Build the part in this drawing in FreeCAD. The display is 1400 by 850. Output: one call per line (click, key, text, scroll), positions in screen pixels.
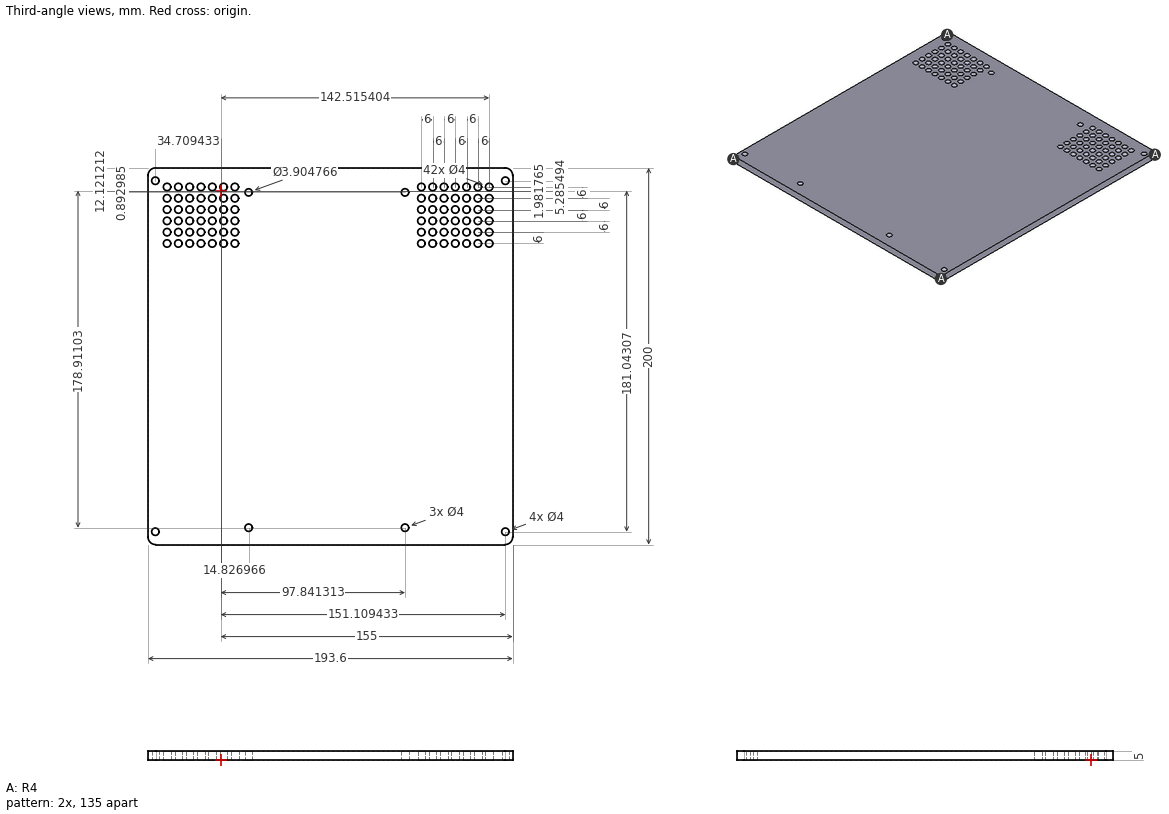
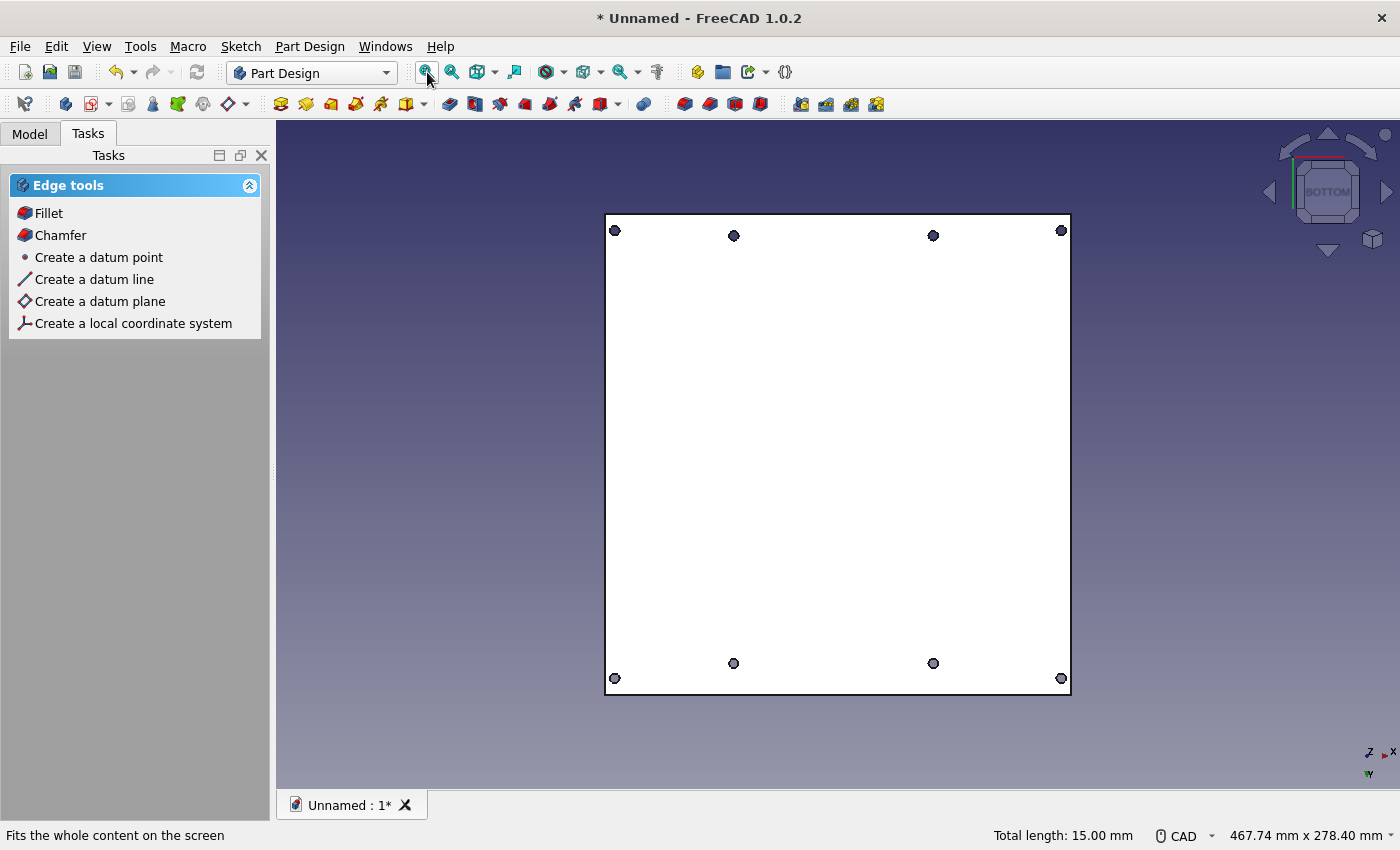
key(4)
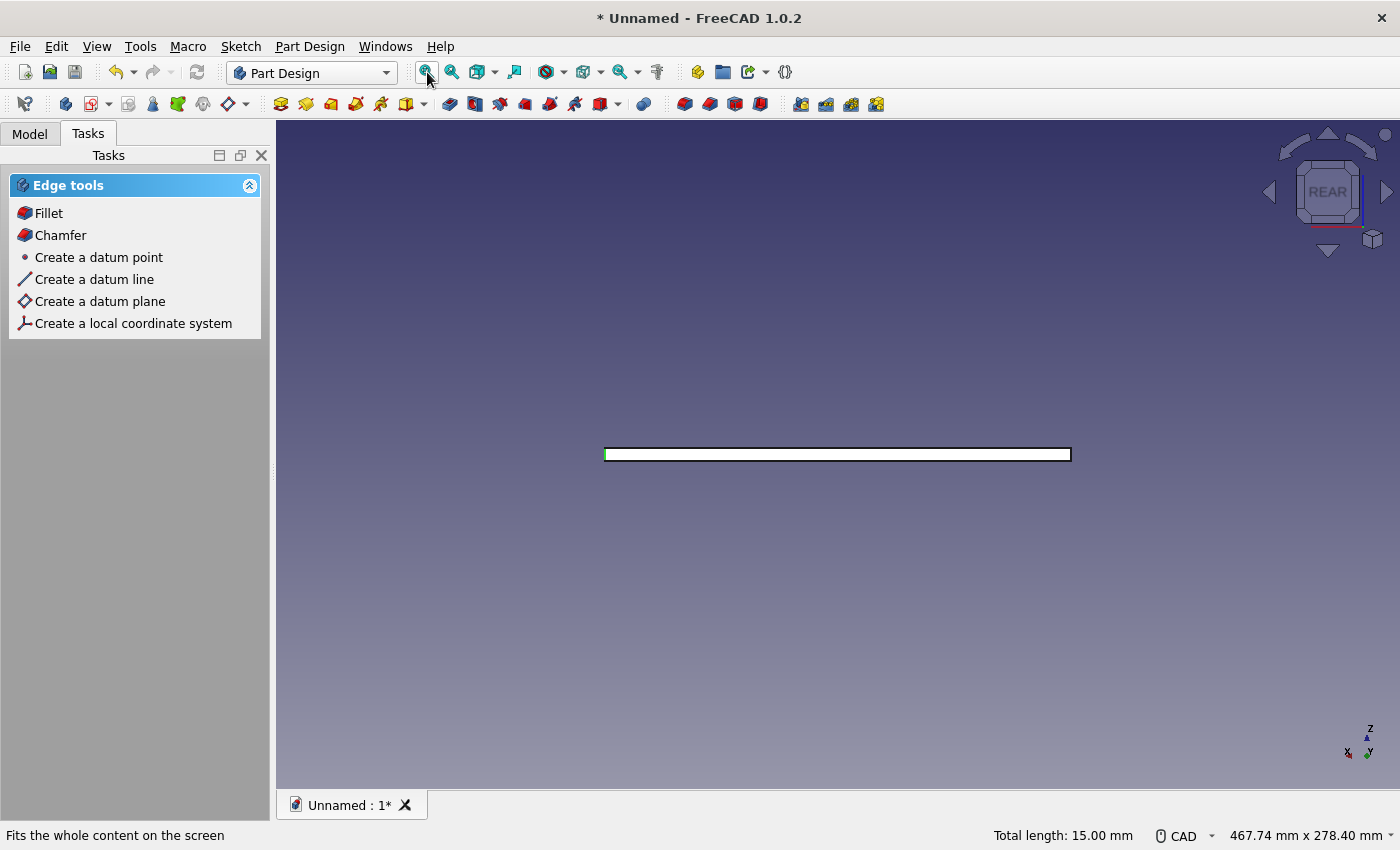
click(427, 72)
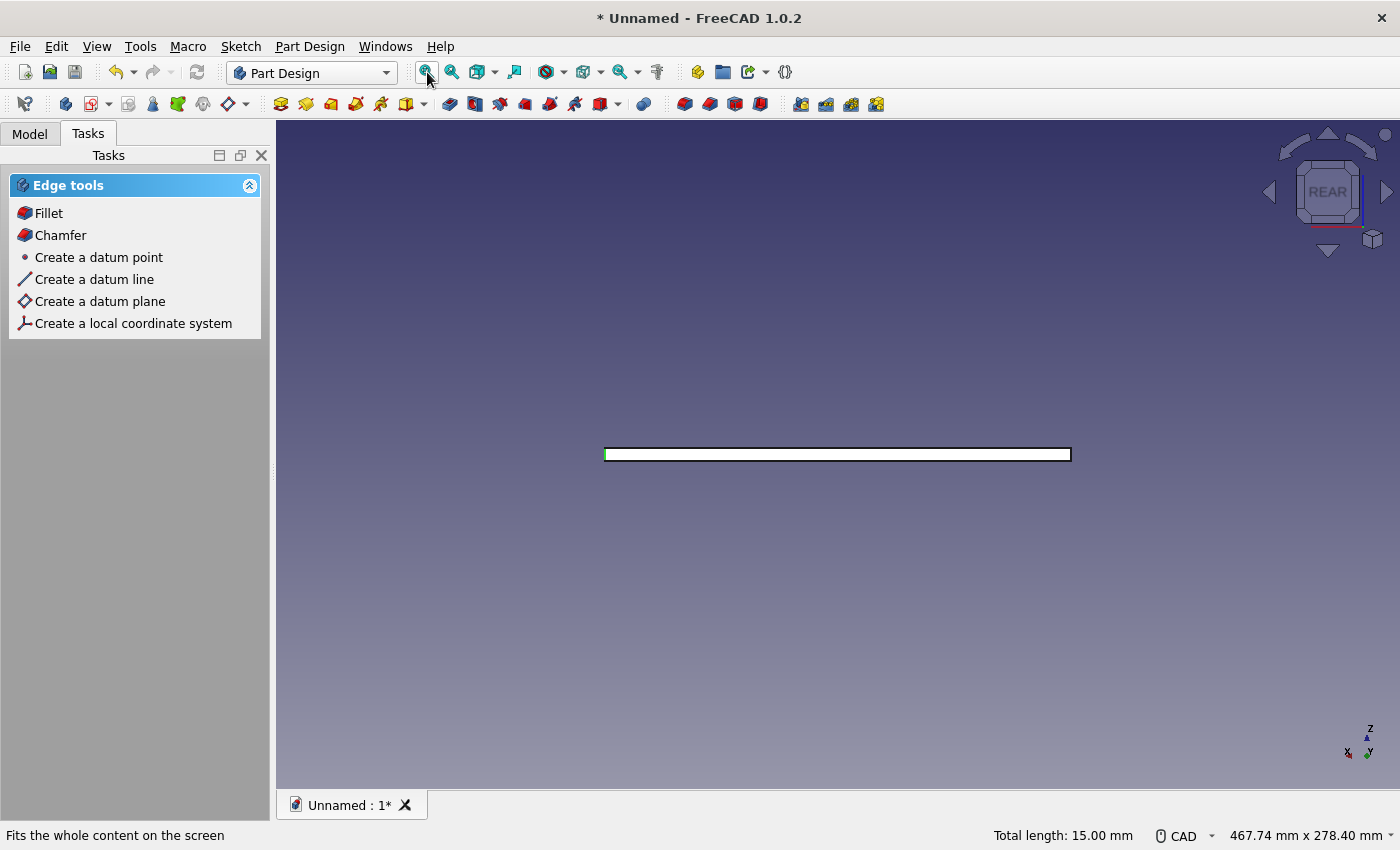
scroll(1071, 454, up, 7)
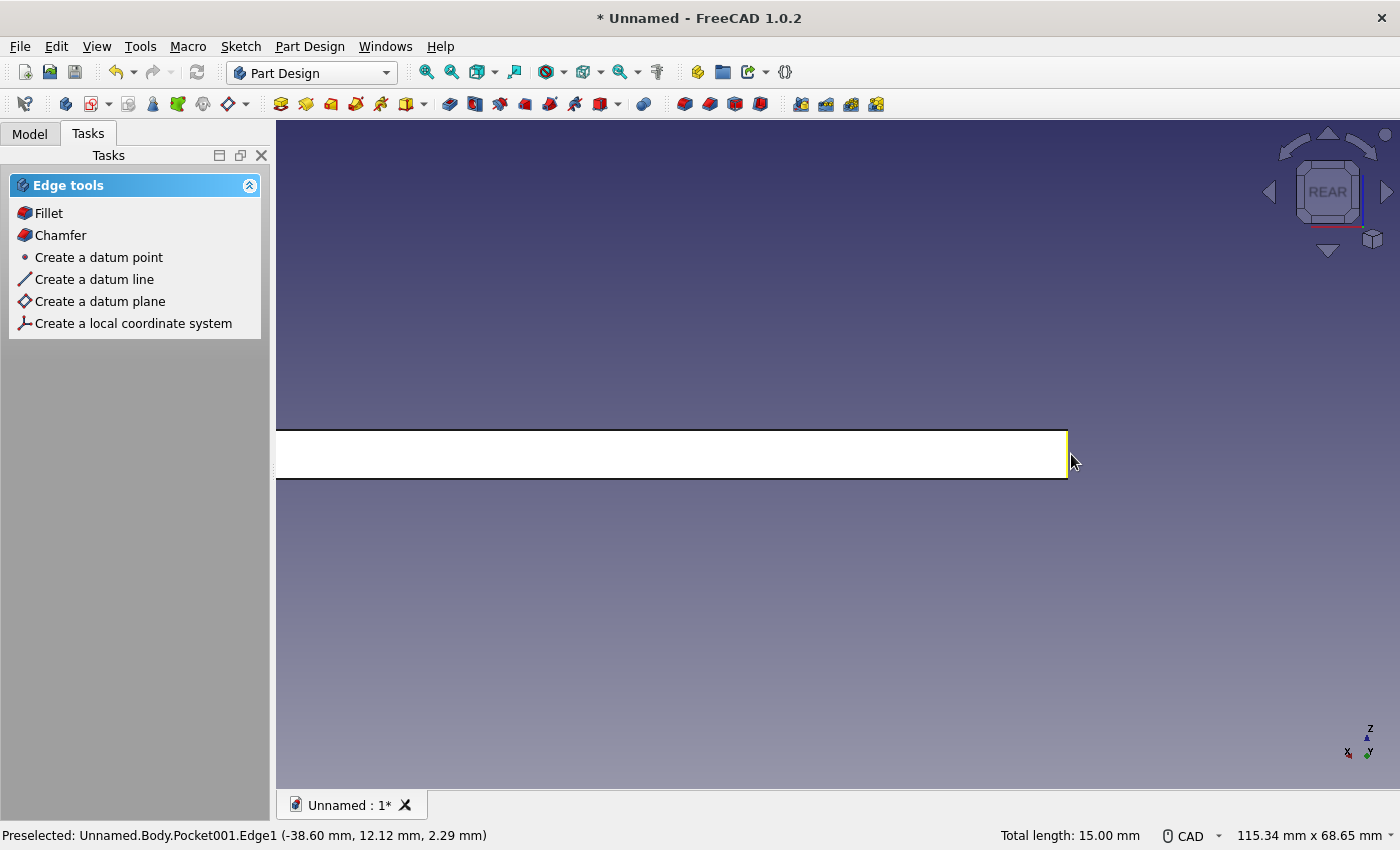
click(1067, 454, ctrl)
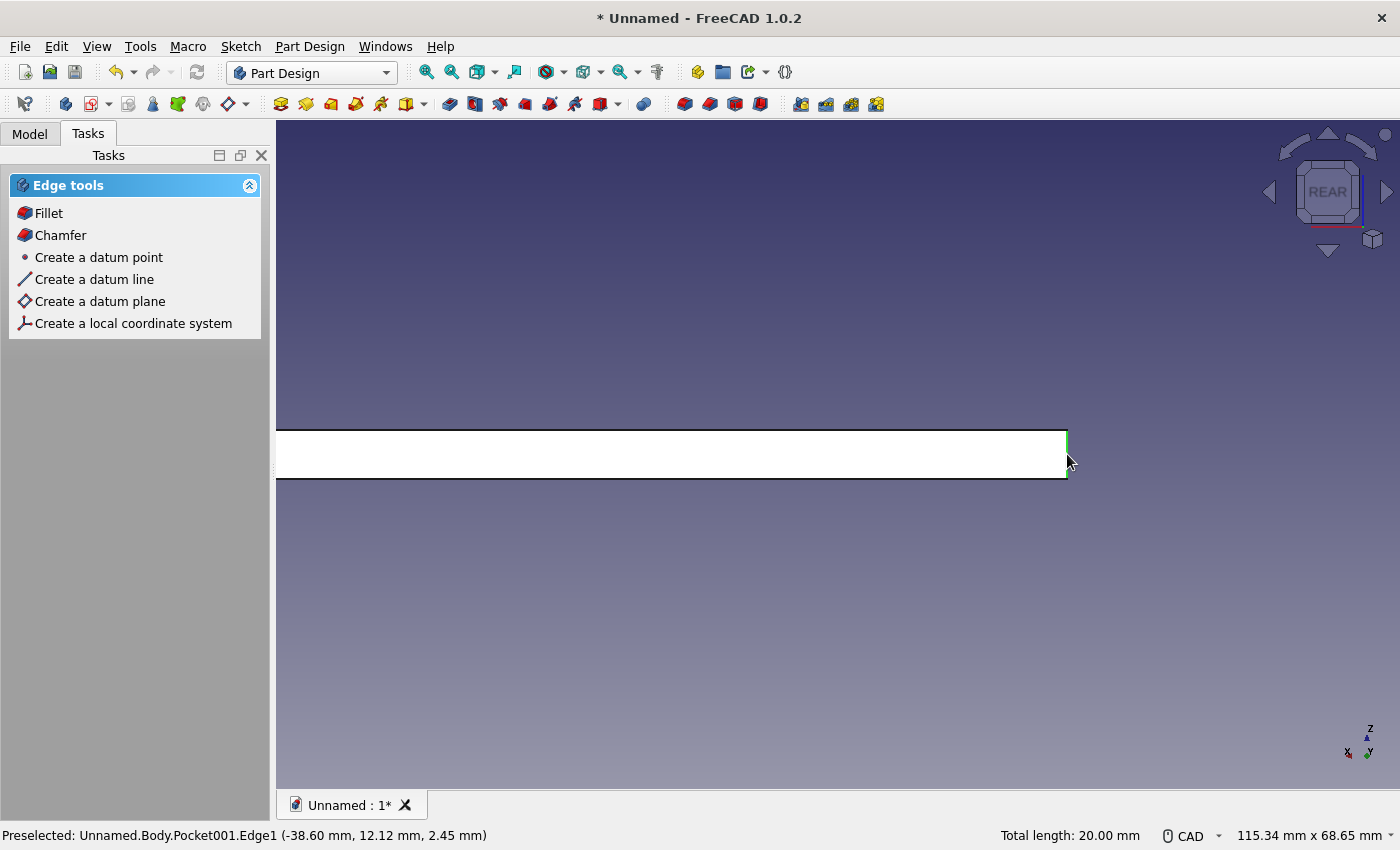
click(685, 104)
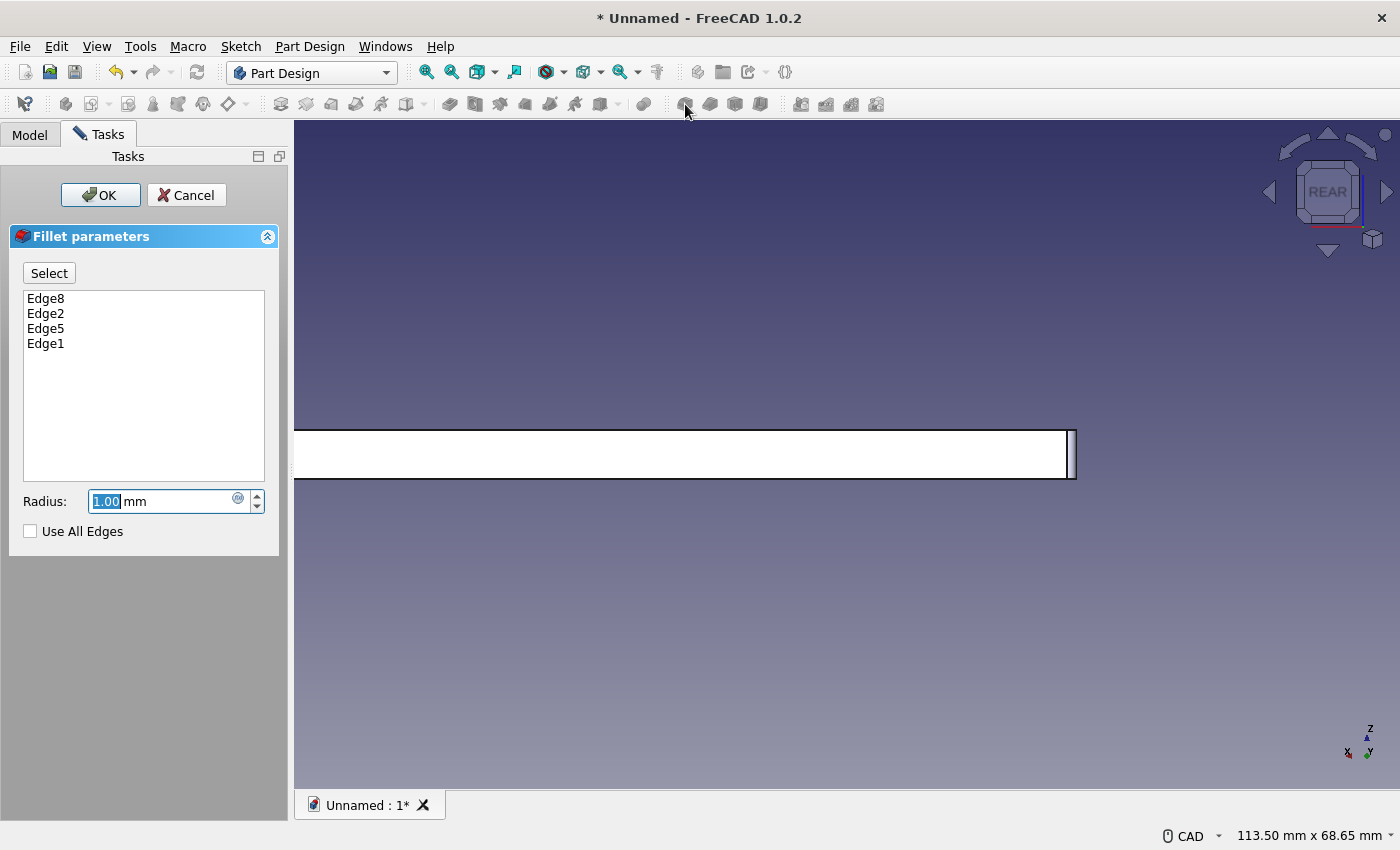
text(4)
key(Tab)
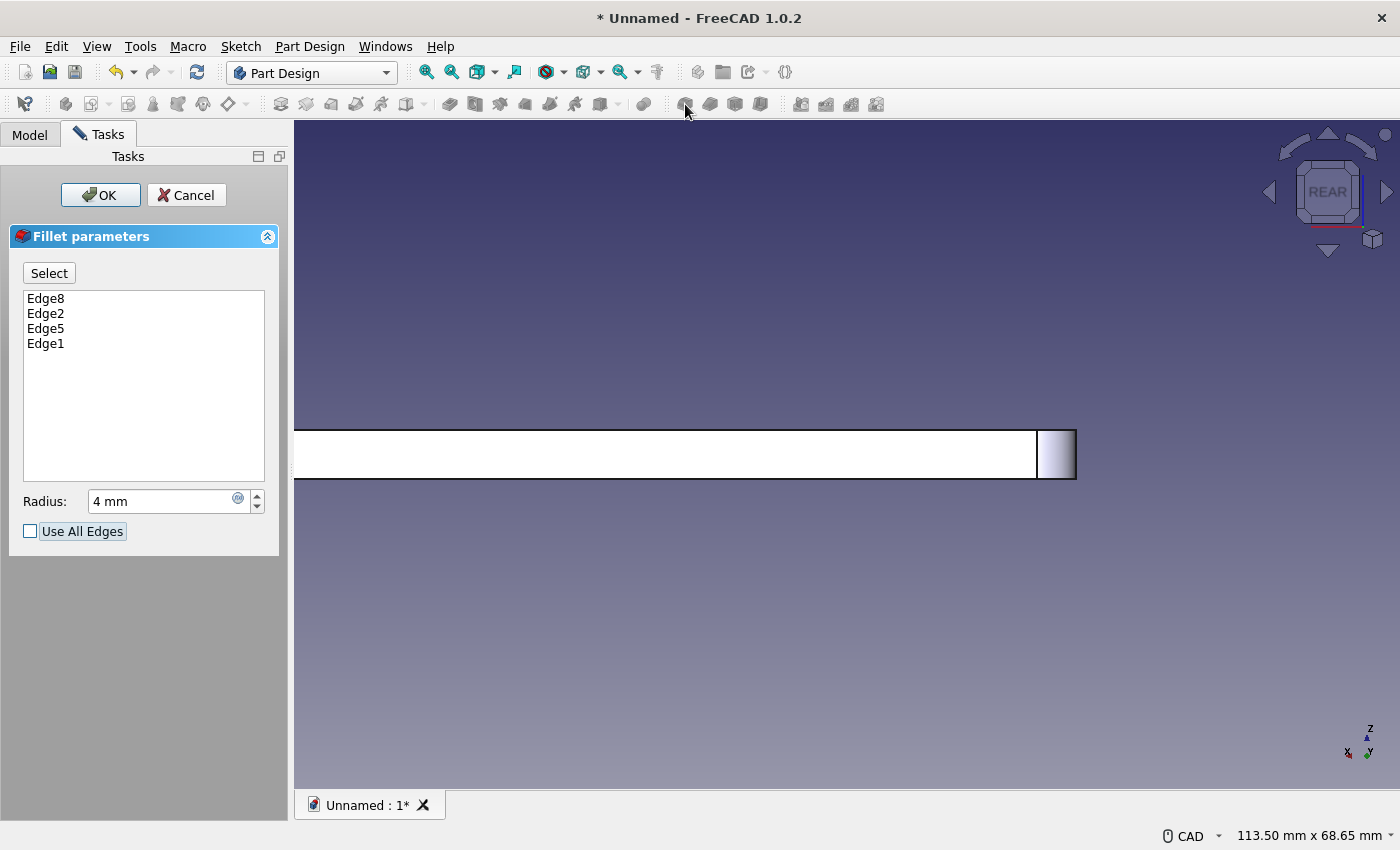
click(101, 195)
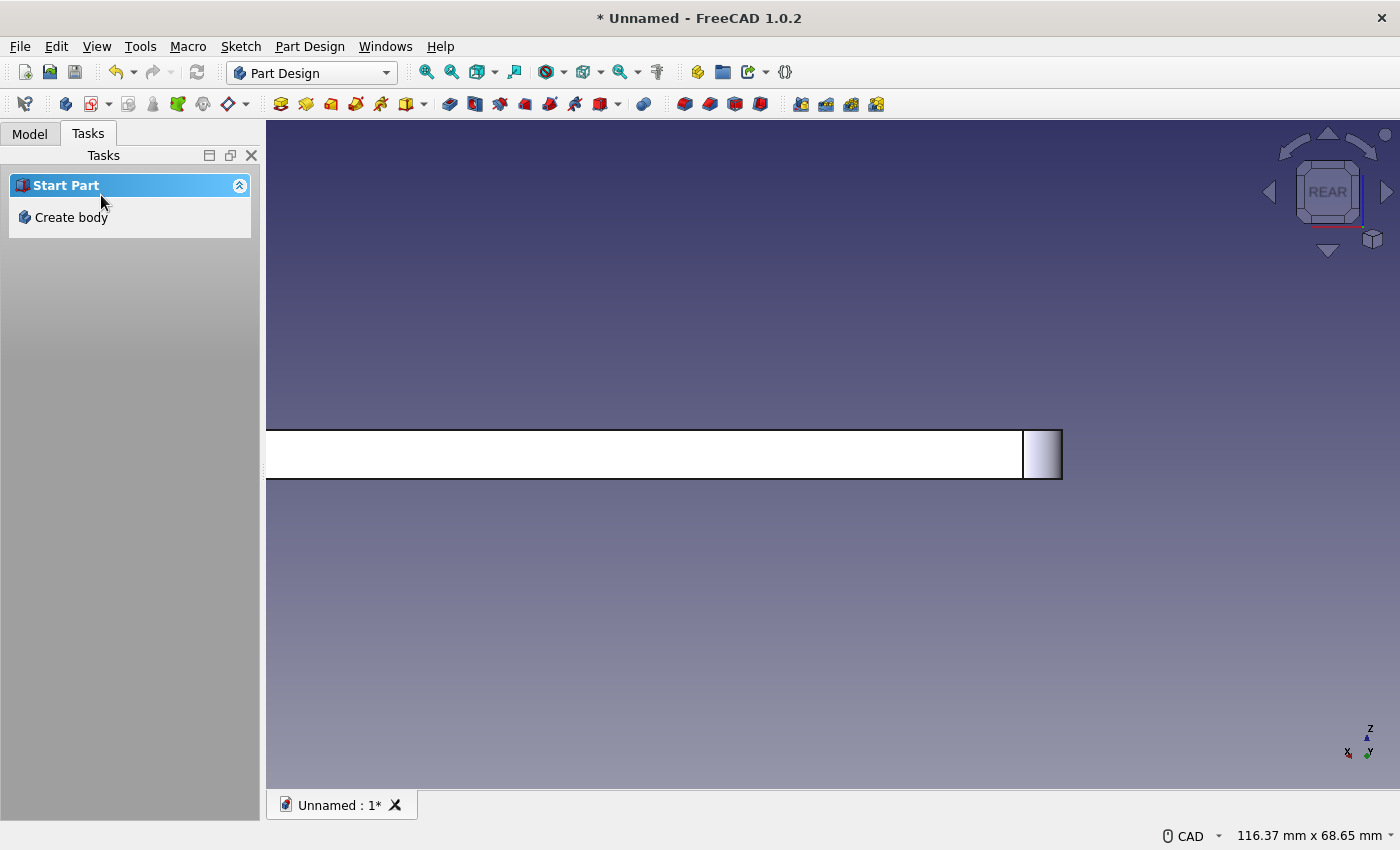
click(427, 72)